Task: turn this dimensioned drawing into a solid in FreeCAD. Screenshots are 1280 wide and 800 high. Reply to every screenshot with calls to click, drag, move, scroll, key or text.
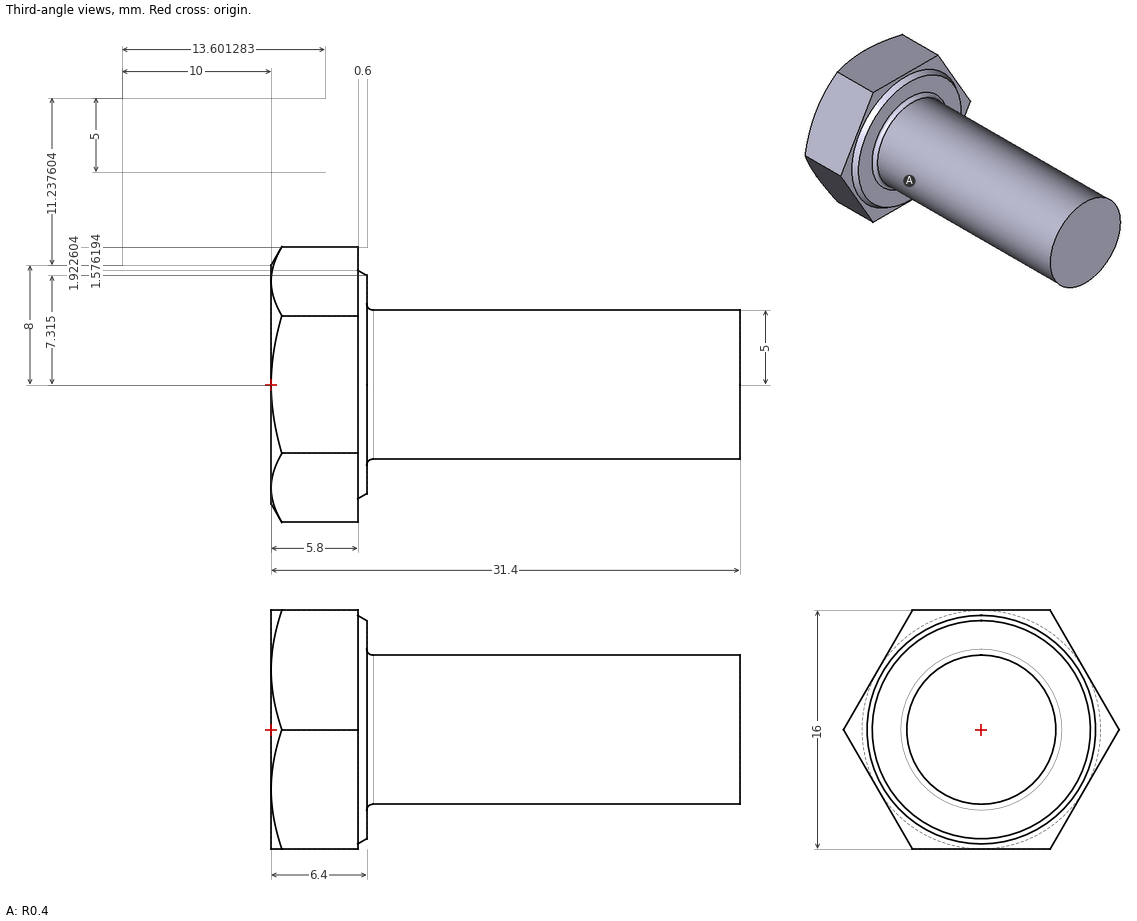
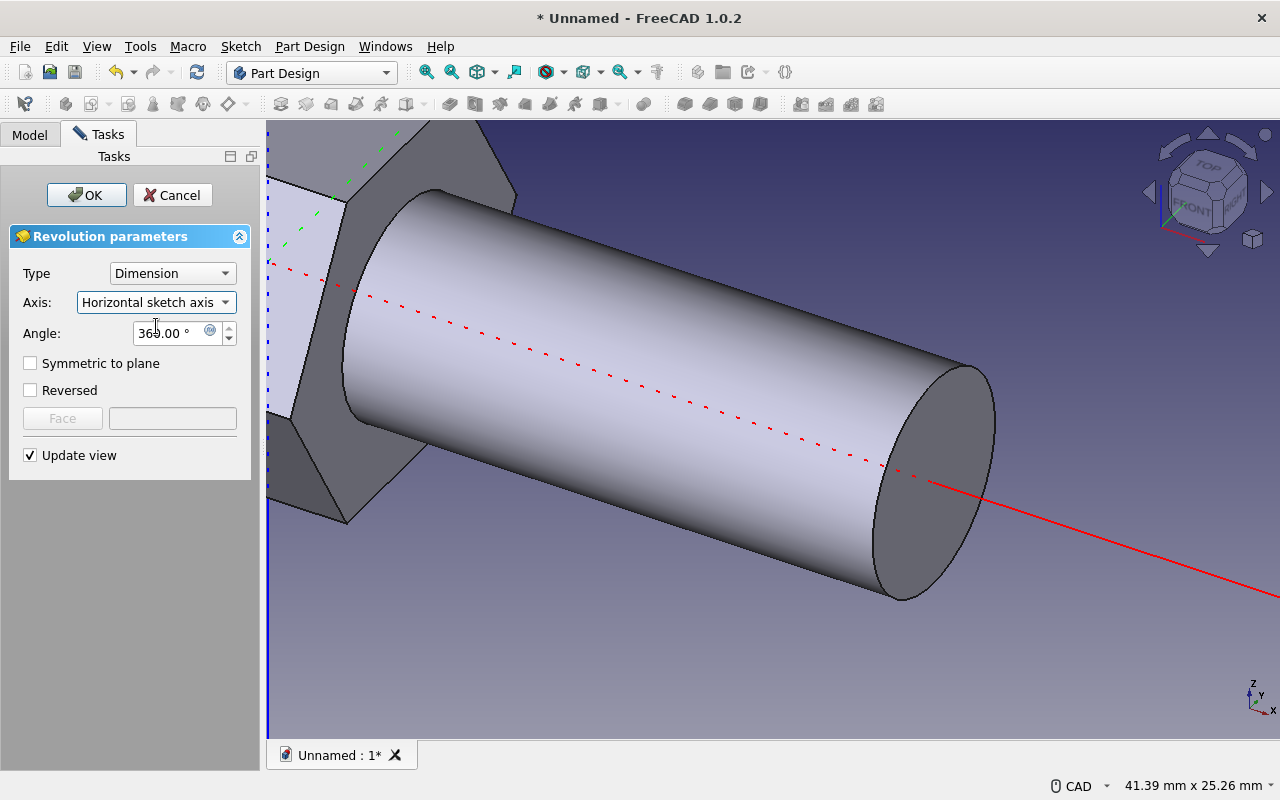
click(87, 195)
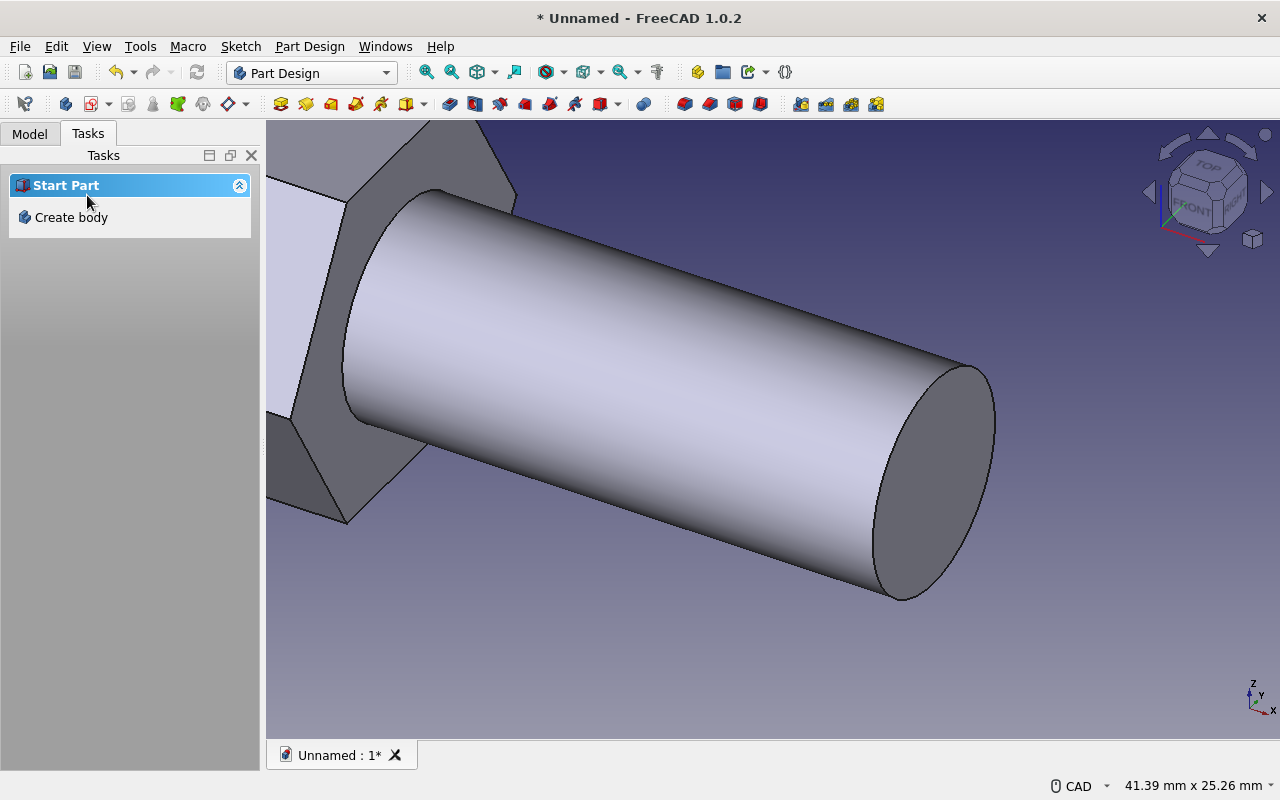
click(427, 72)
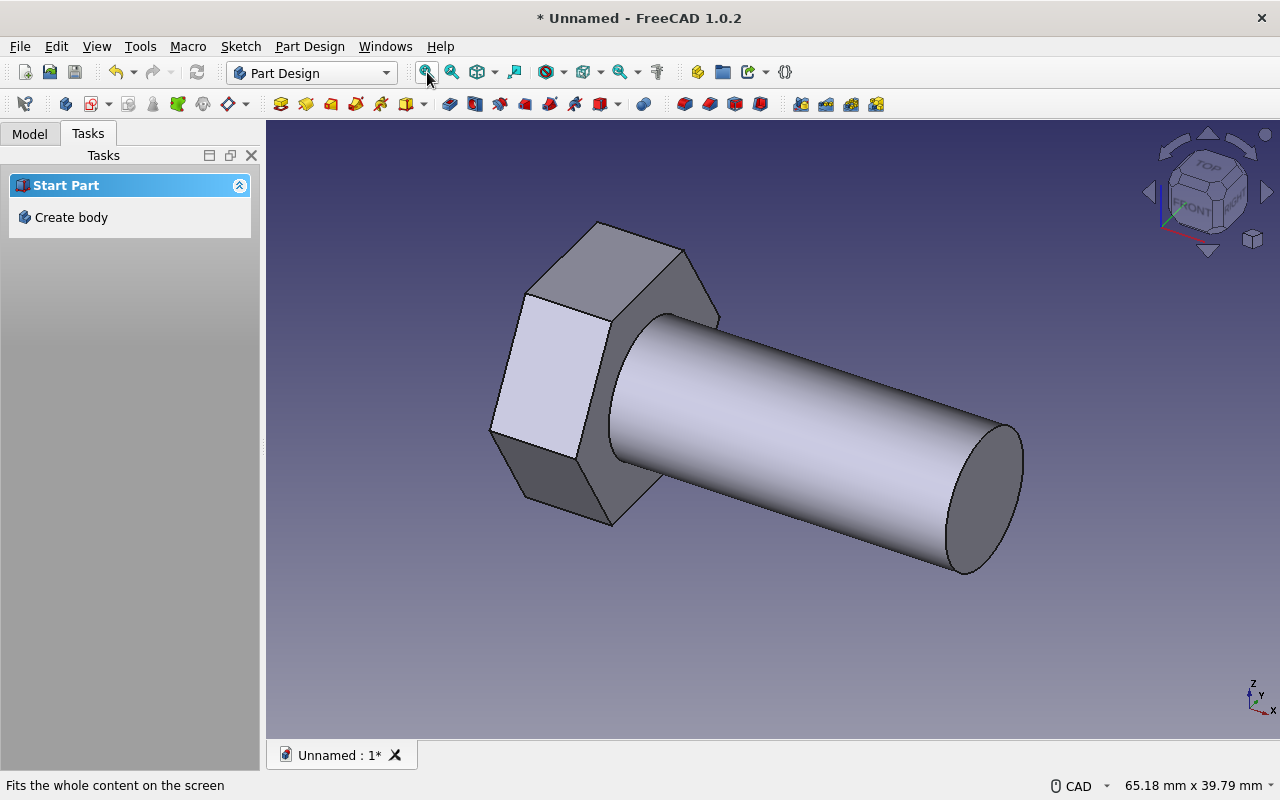
click(90, 104)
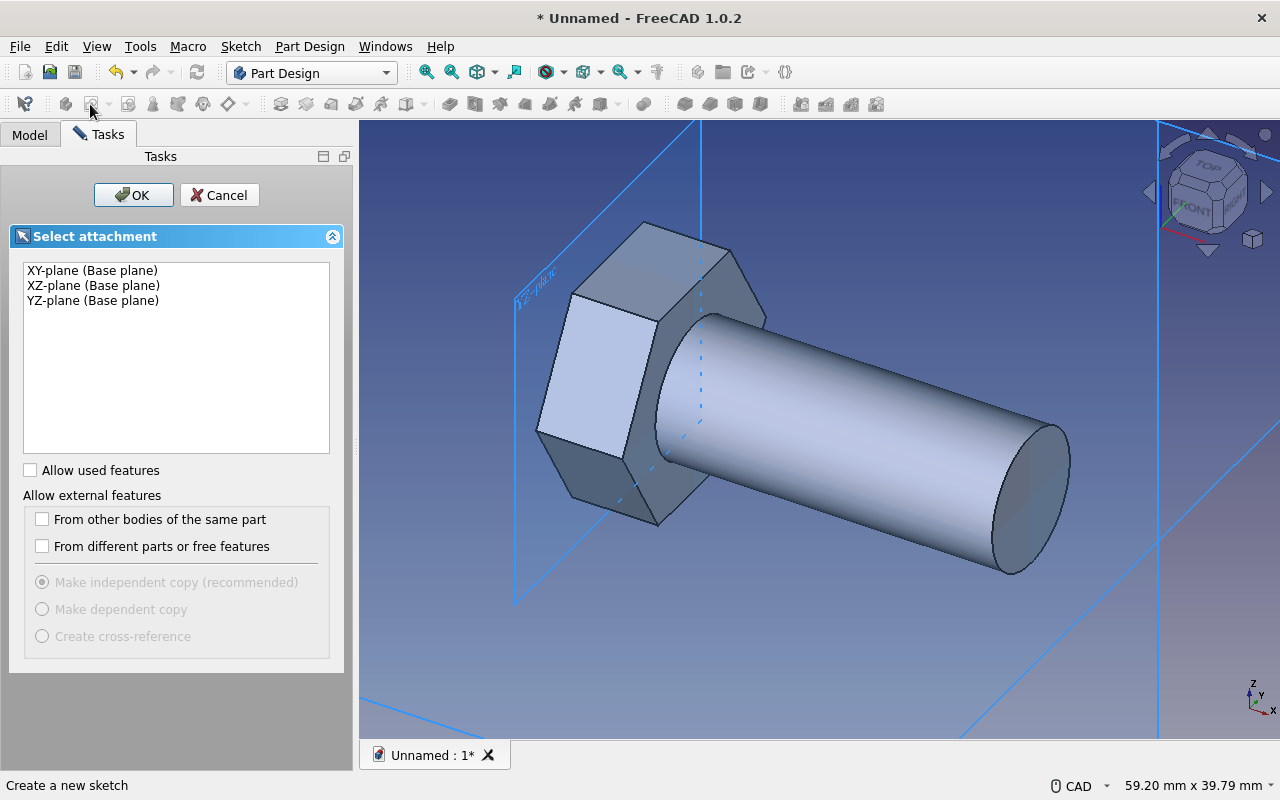
click(84, 270)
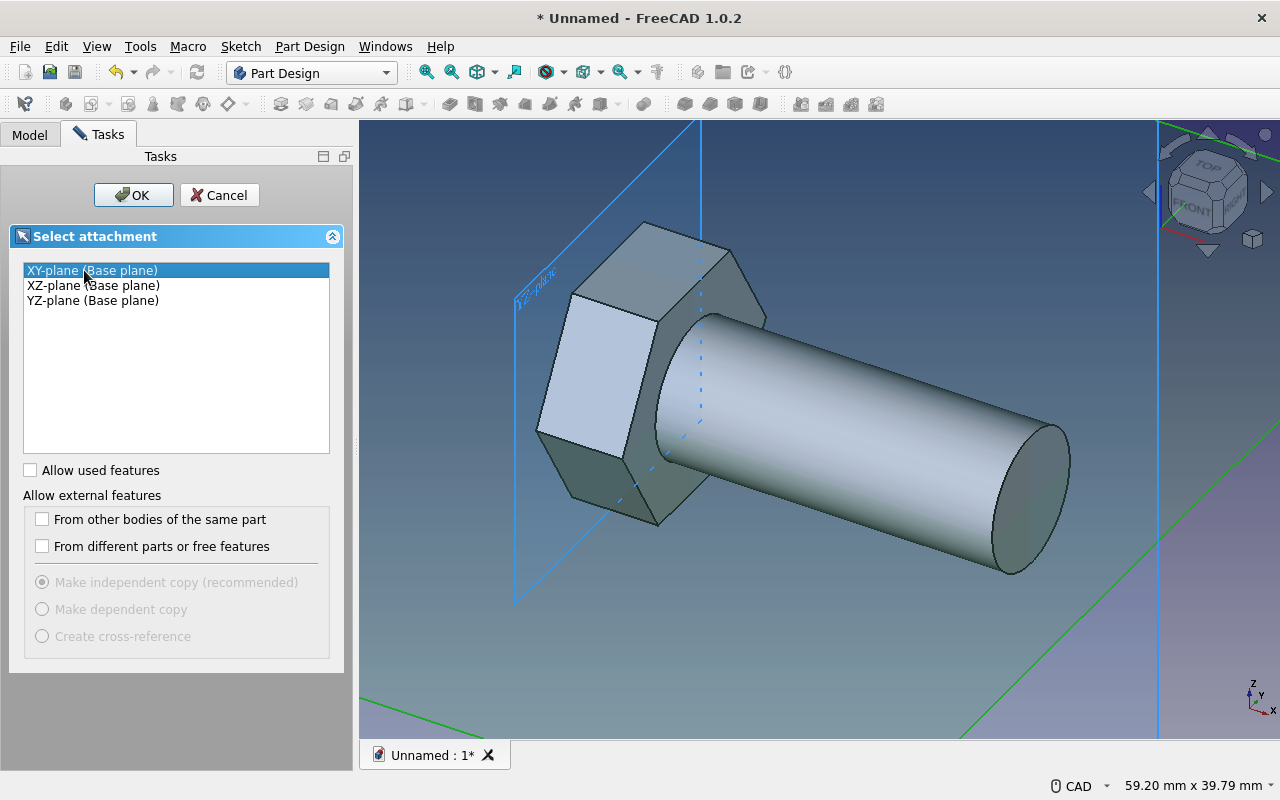
click(134, 195)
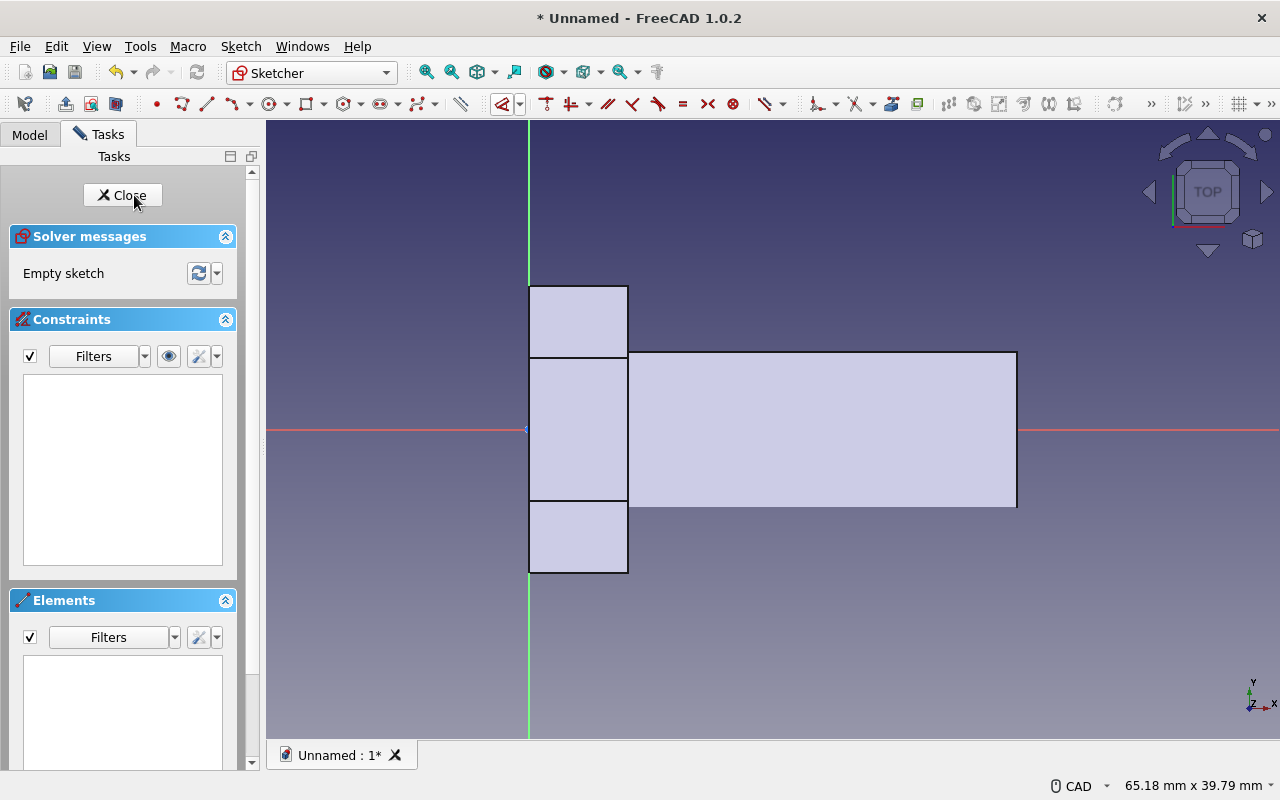
click(116, 104)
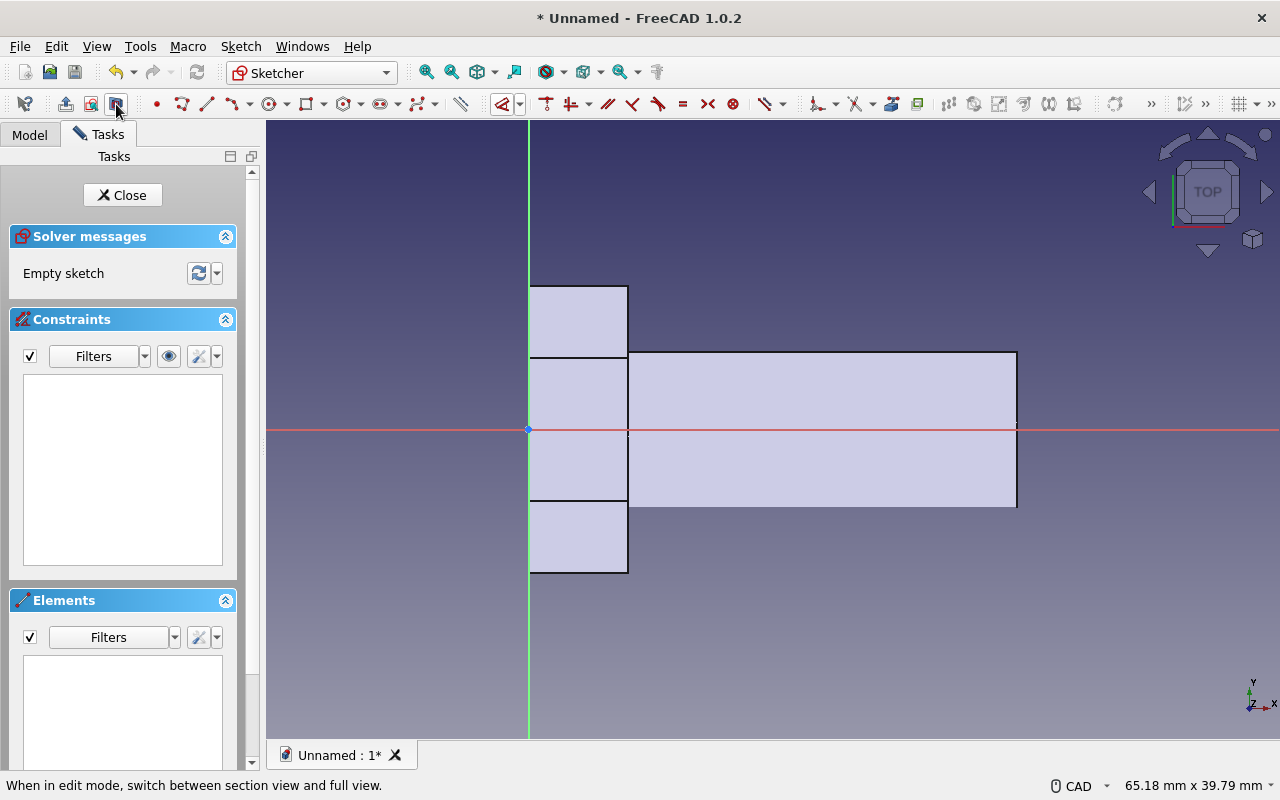
scroll(1115, 711, down, 1)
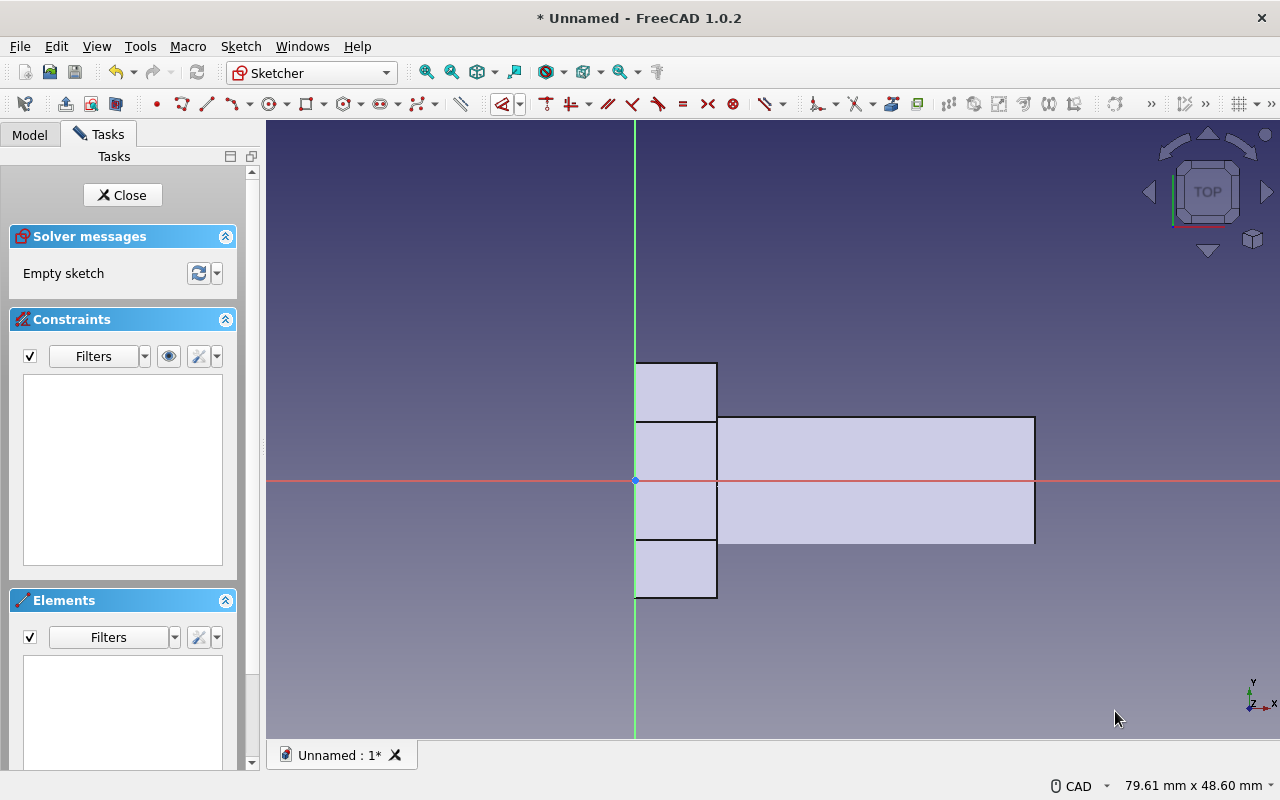
scroll(371, 213, up, 2)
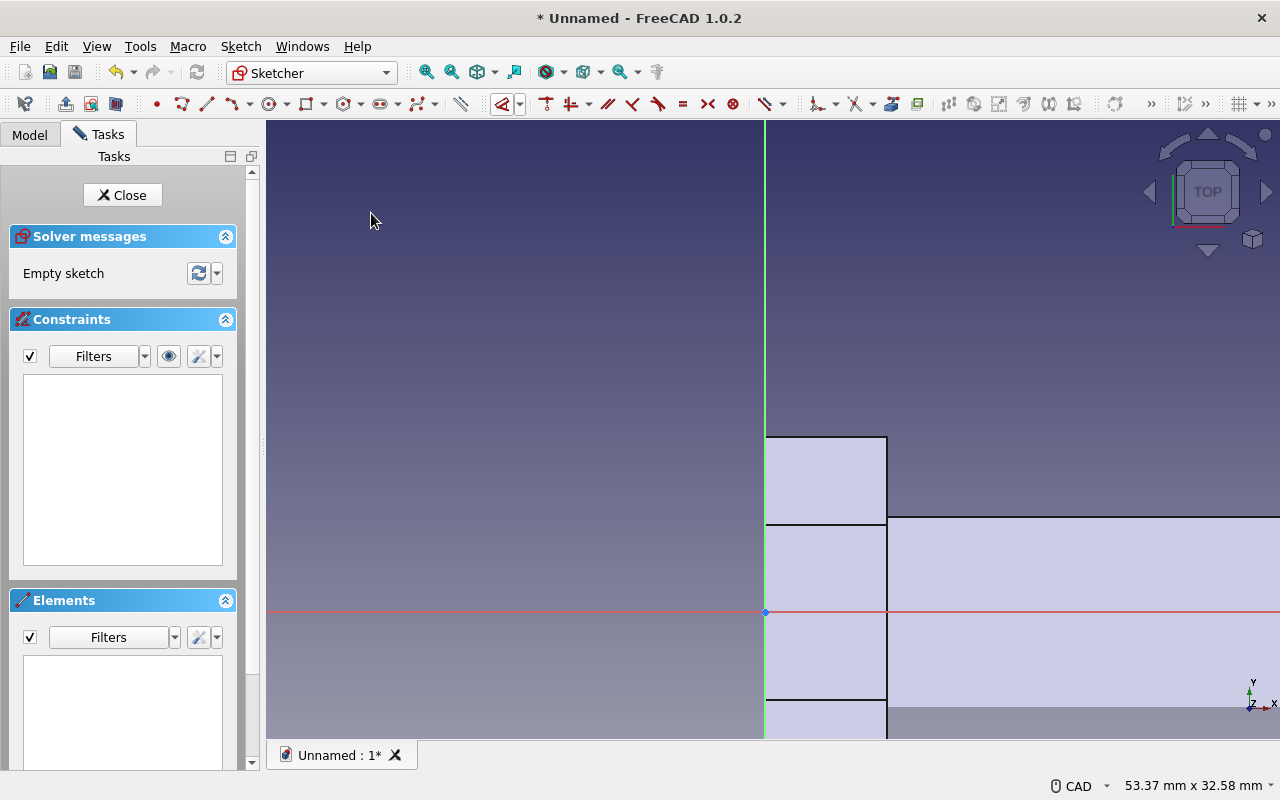
click(182, 104)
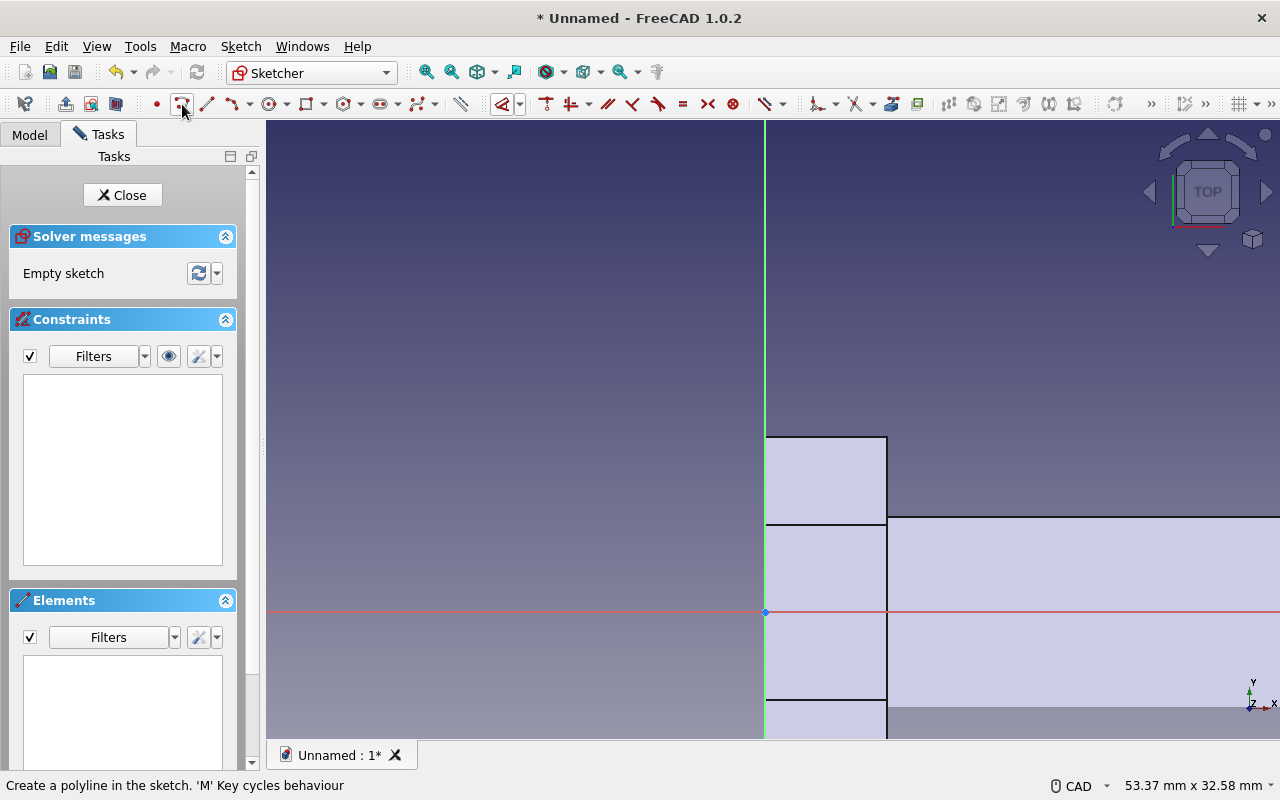
click(765, 460)
click(833, 342)
click(833, 247)
click(575, 247)
click(575, 460)
click(765, 461)
key(Escape)
key(Escape)